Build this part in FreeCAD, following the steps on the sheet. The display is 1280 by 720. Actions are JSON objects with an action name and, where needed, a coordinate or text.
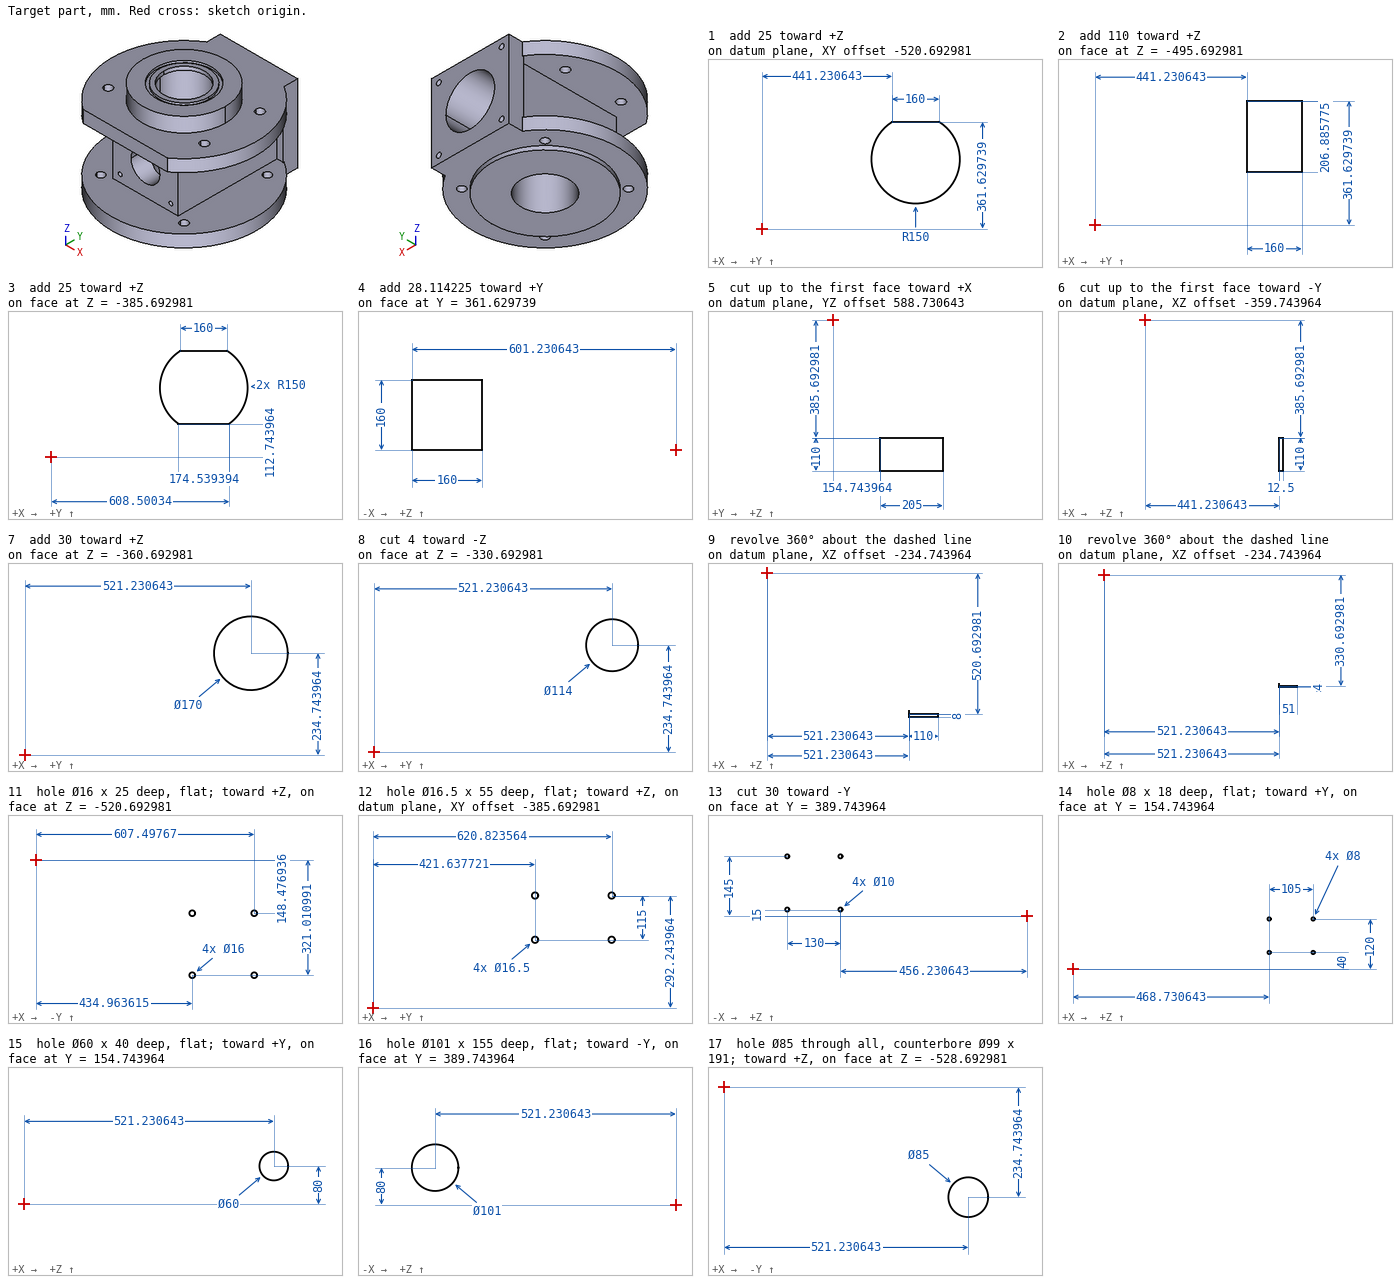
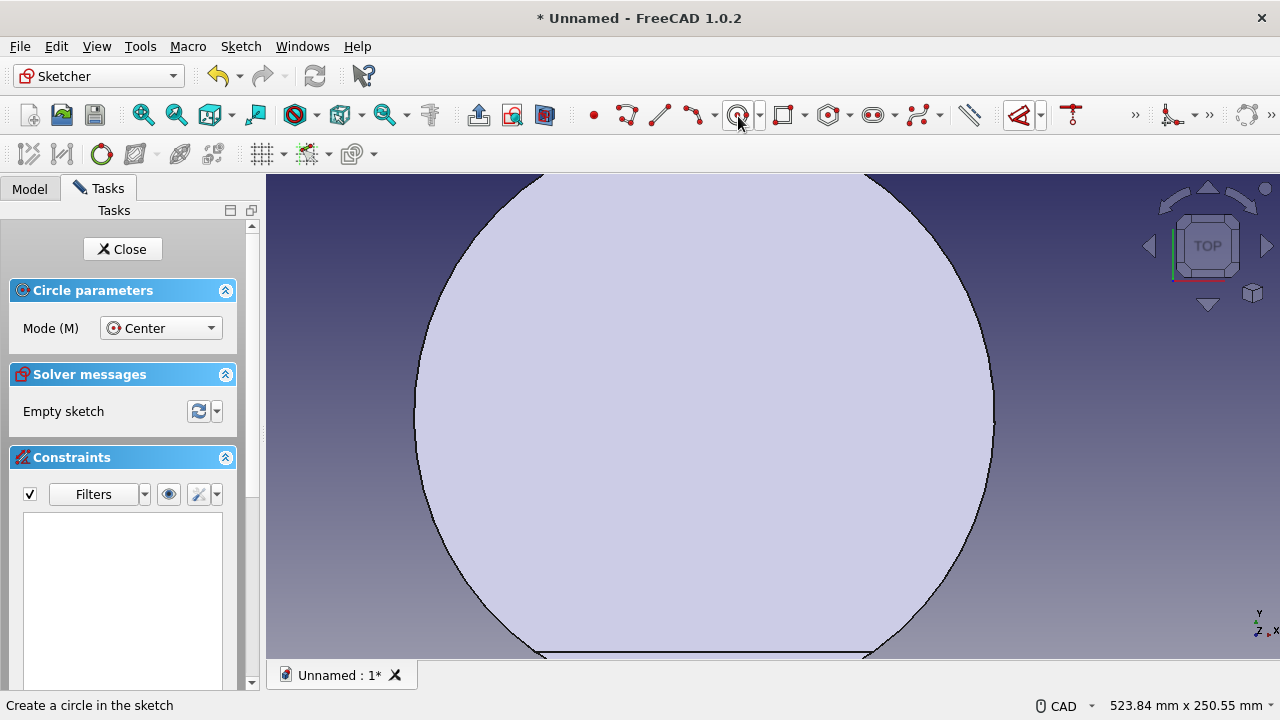
{"action": "left_click", "coordinate": [704, 416]}
{"action": "left_click", "coordinate": [821, 299]}
{"action": "key", "text": "Escape"}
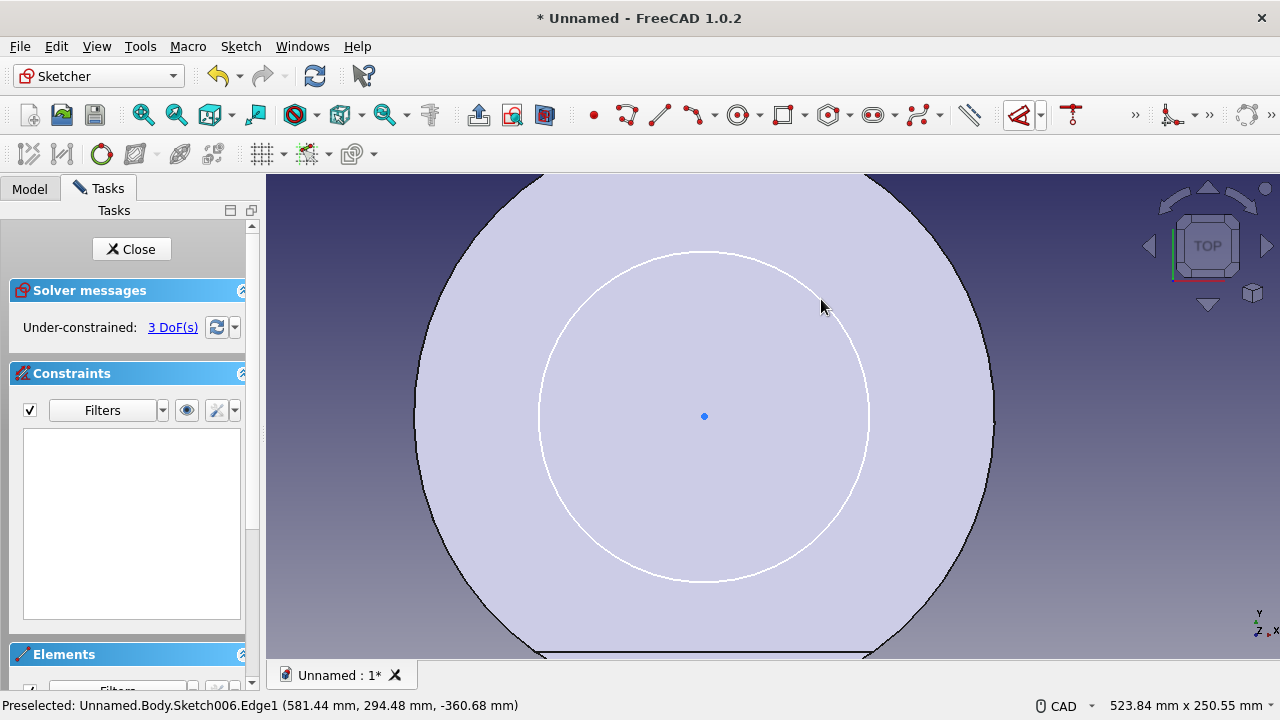
{"action": "left_click", "coordinate": [821, 300]}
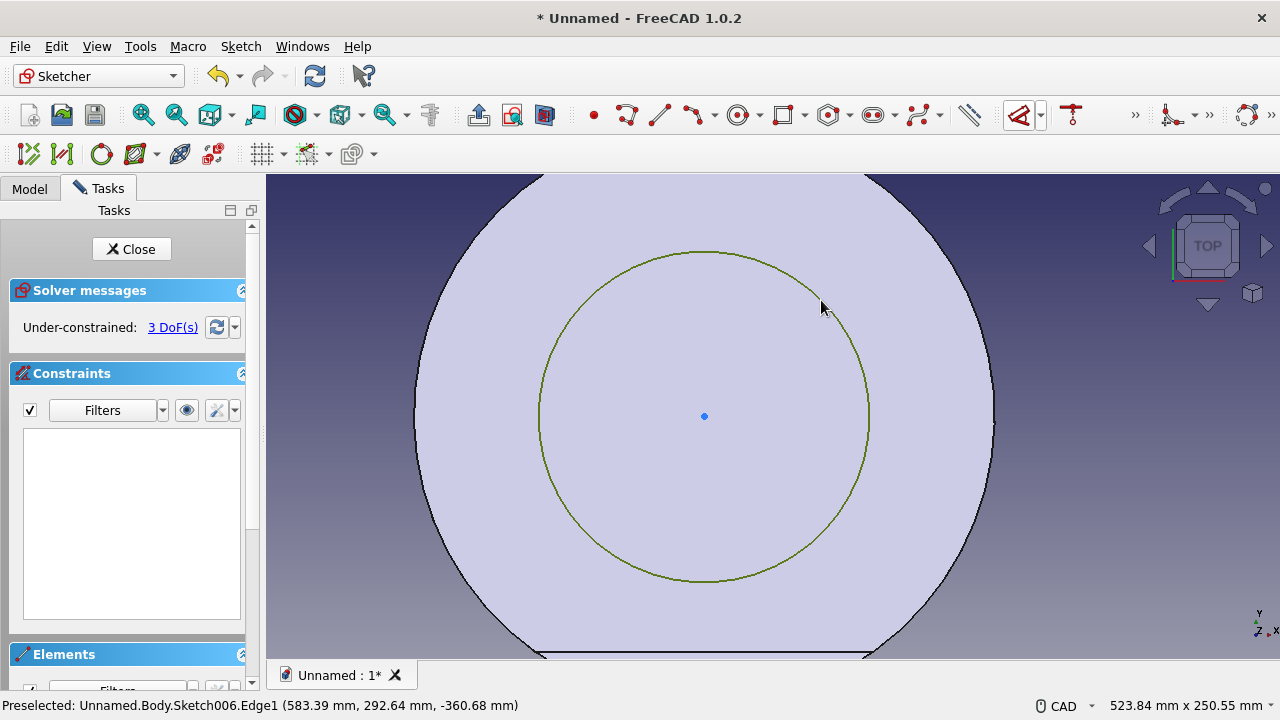
{"action": "key", "text": "k o"}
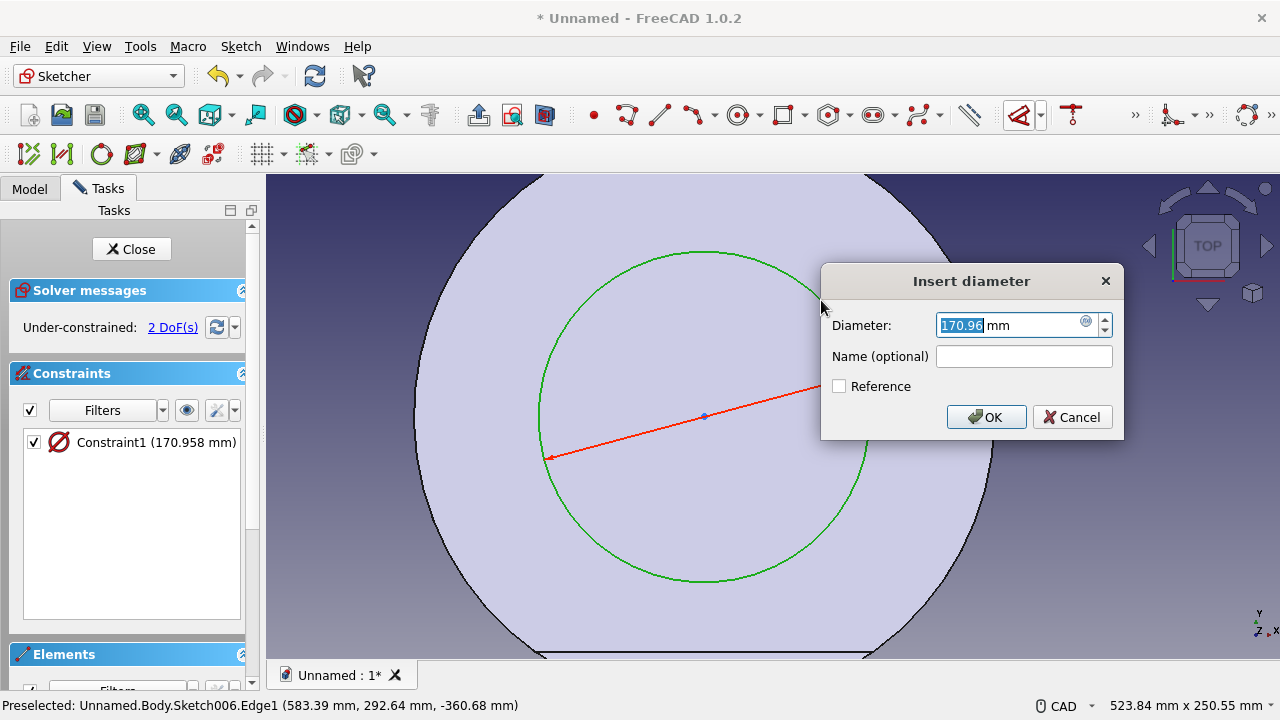
{"action": "type", "text": "170"}
{"action": "key", "text": "Return"}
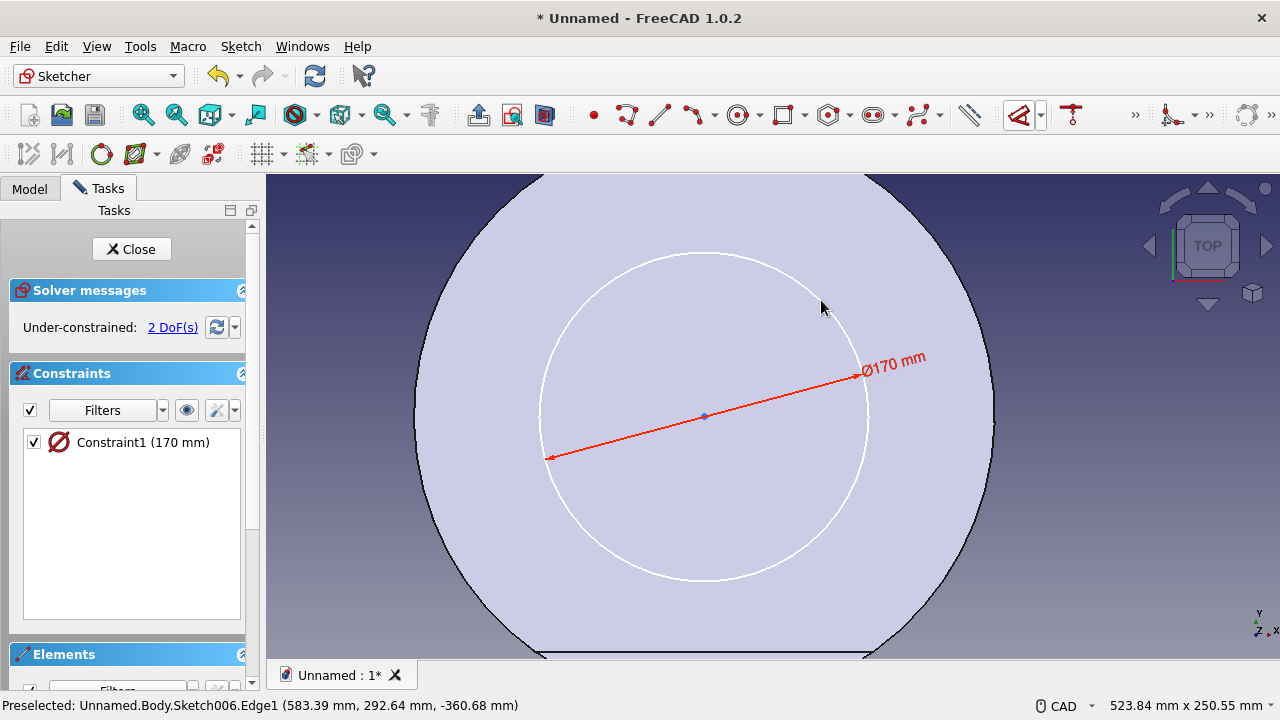
{"action": "left_click", "coordinate": [704, 417]}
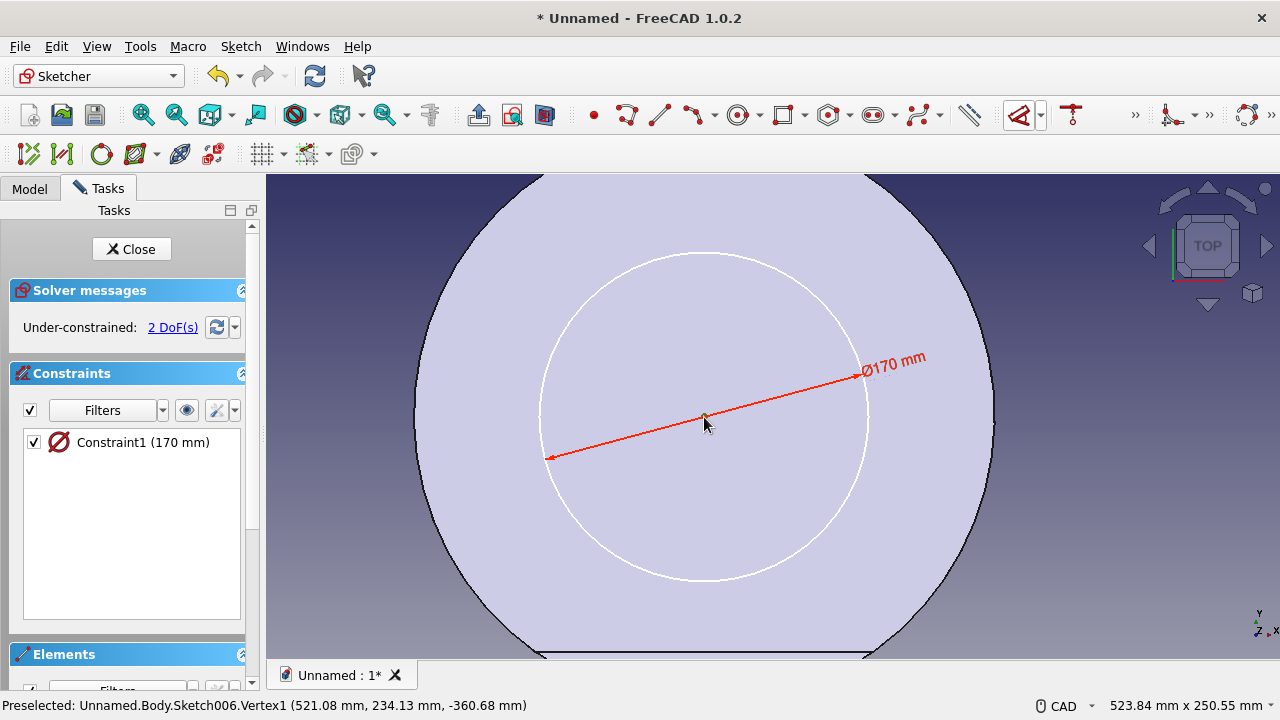
{"action": "key", "text": "l"}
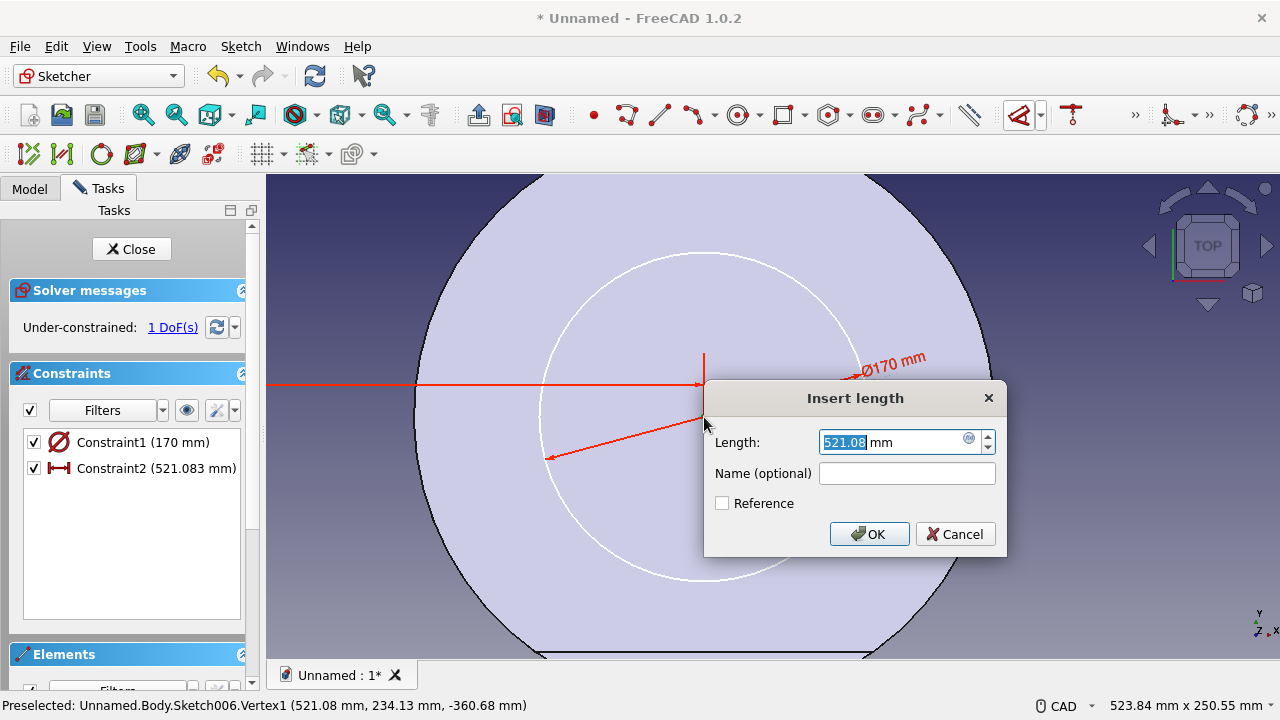
{"action": "type", "text": "521.230643"}
{"action": "key", "text": "Return"}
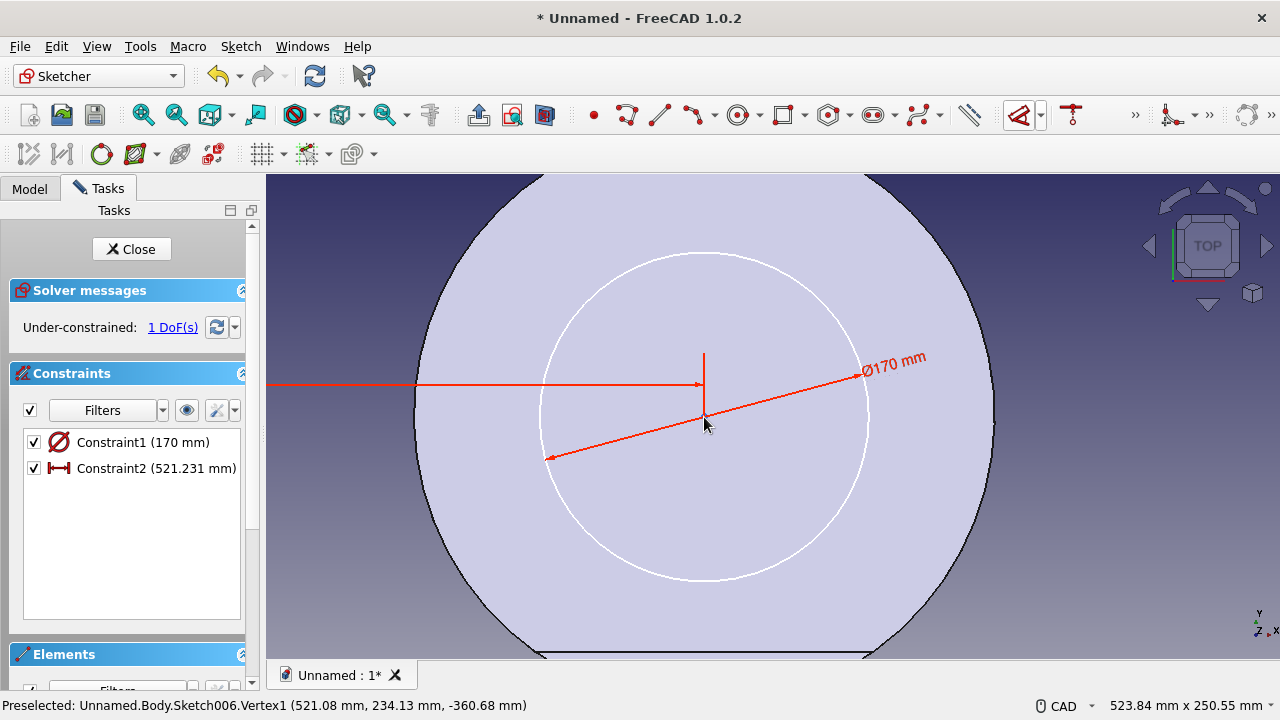
{"action": "left_click", "coordinate": [704, 417]}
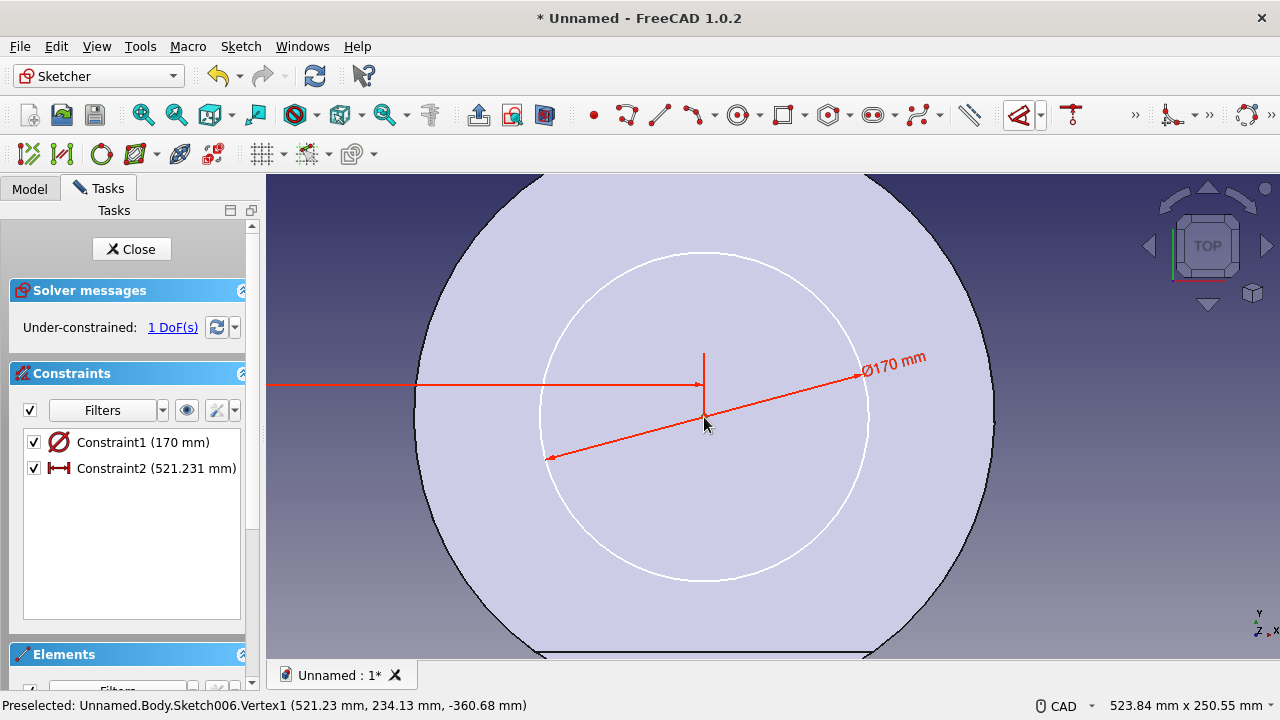
{"action": "key", "text": "i"}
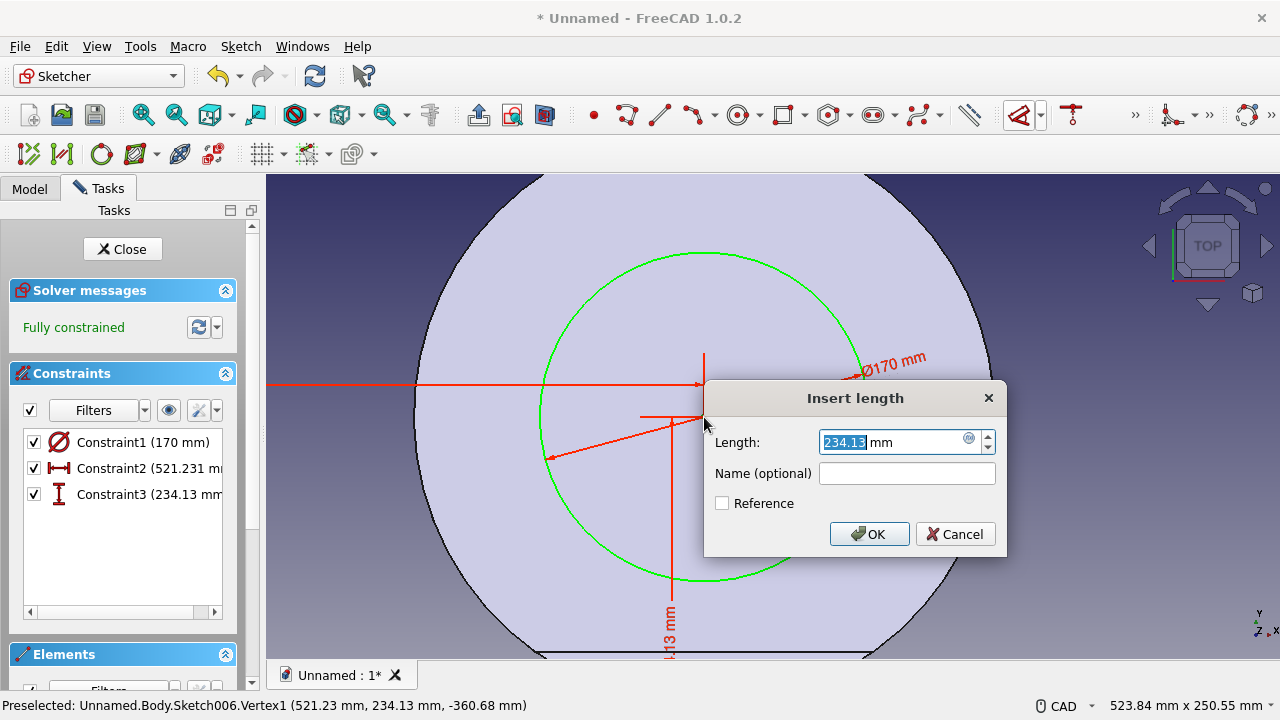
{"action": "type", "text": "234.743964"}
{"action": "key", "text": "Return"}